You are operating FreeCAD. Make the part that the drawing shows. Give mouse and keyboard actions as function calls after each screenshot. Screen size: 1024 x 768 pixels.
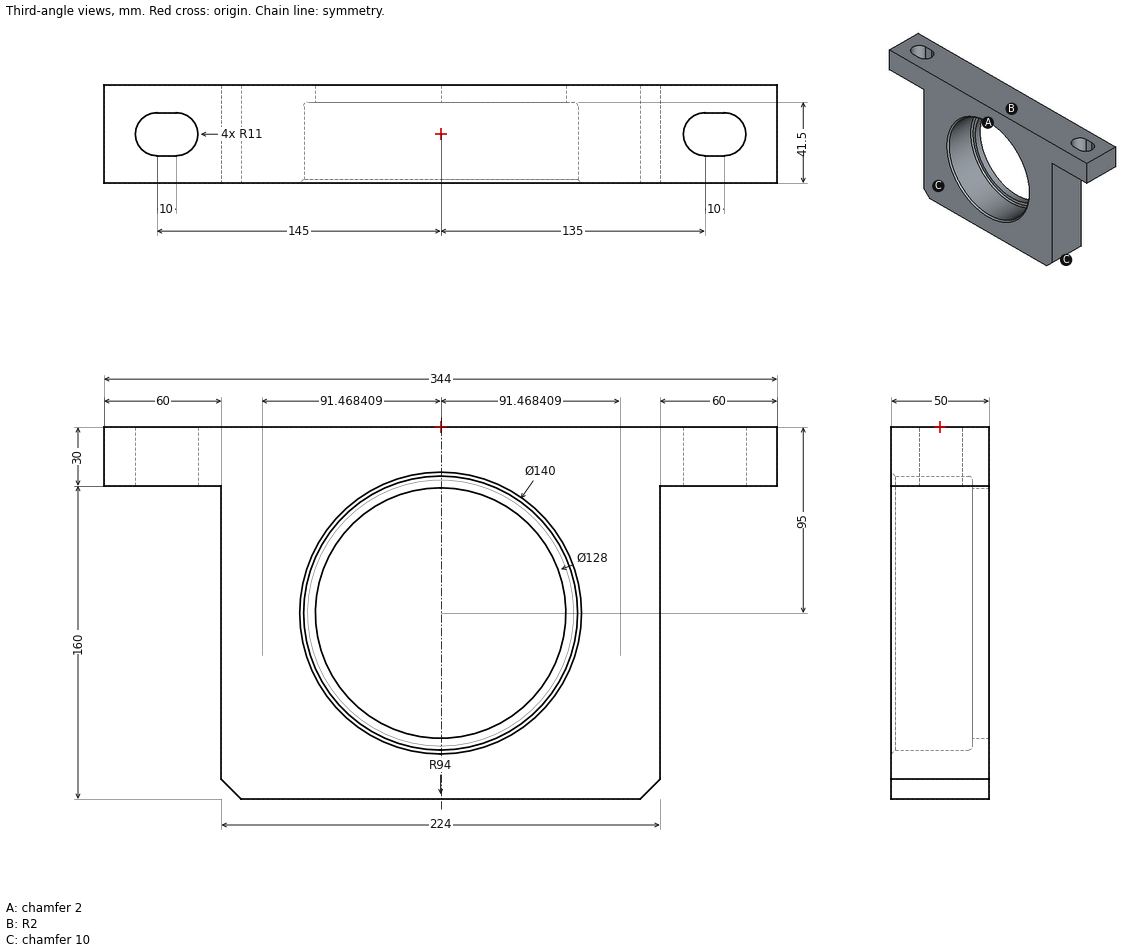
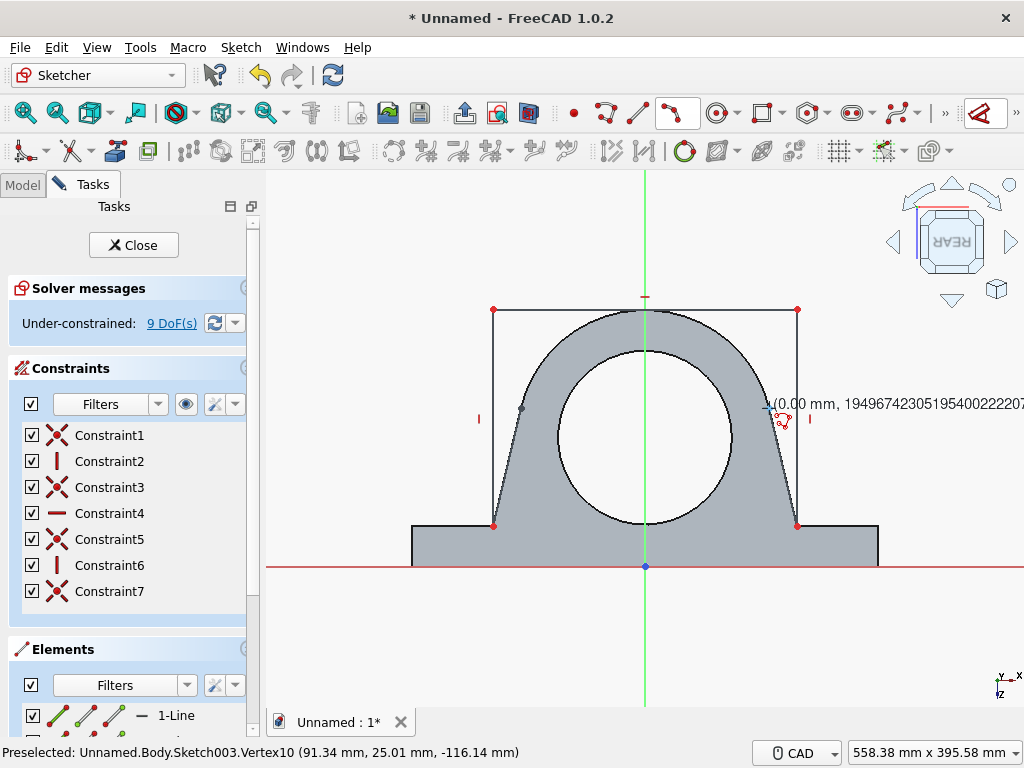
key(g)
key(3)
key(a)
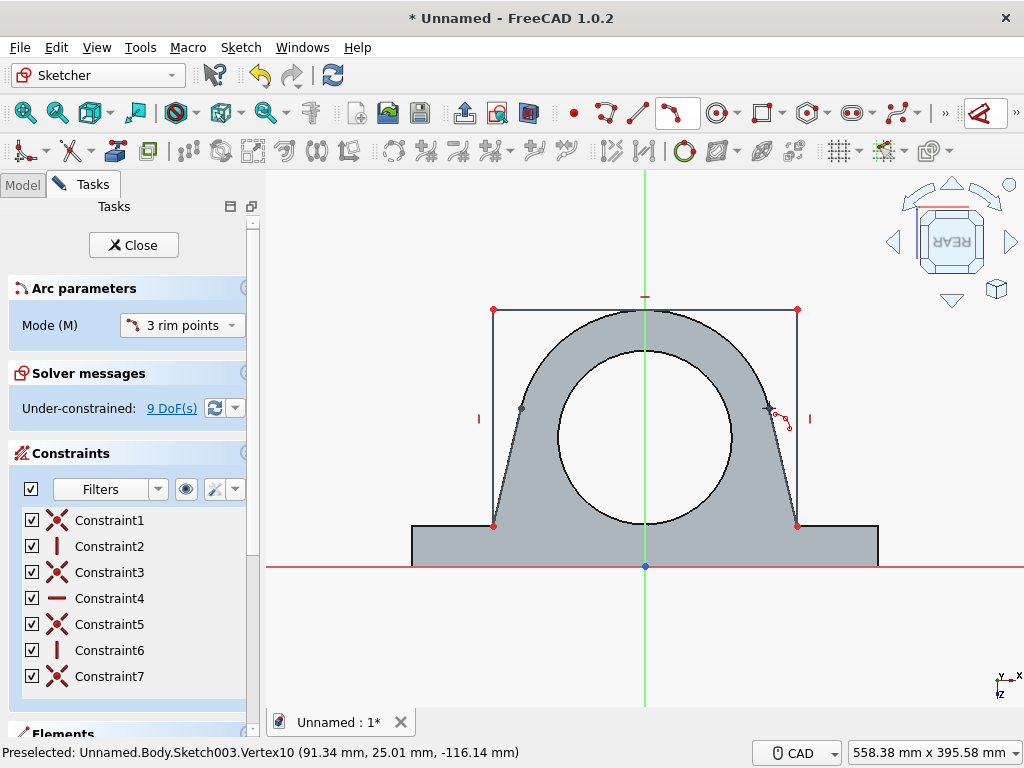
click(769, 409)
click(521, 409)
click(710, 328)
key(Escape)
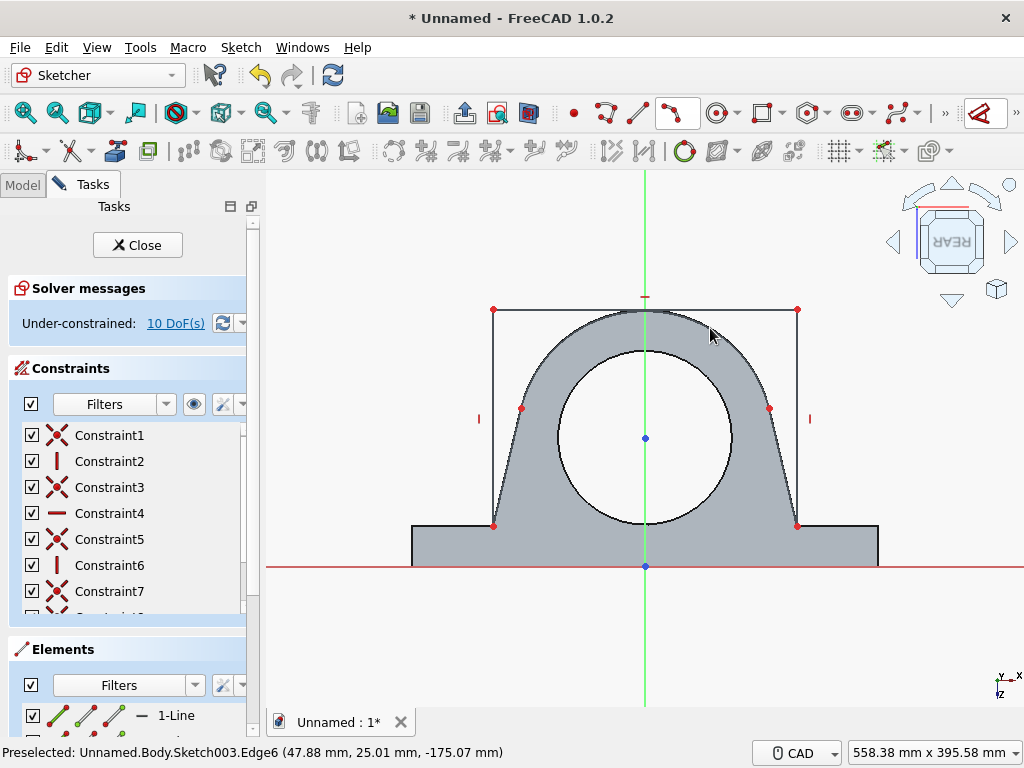
click(645, 439)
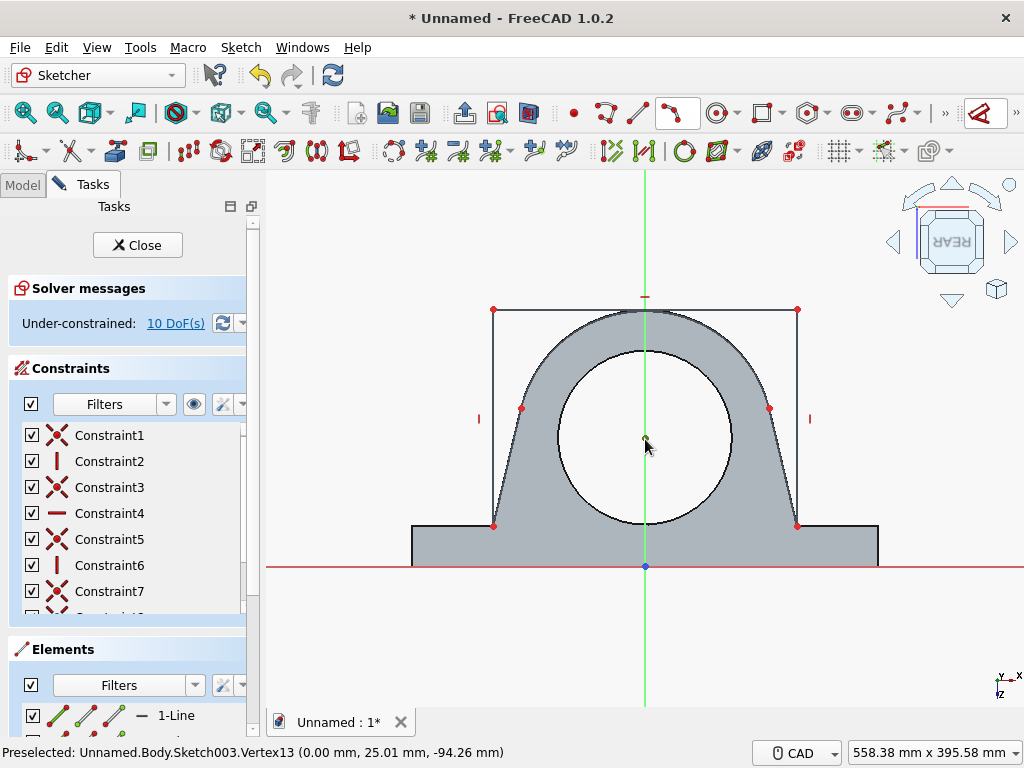
click(645, 645)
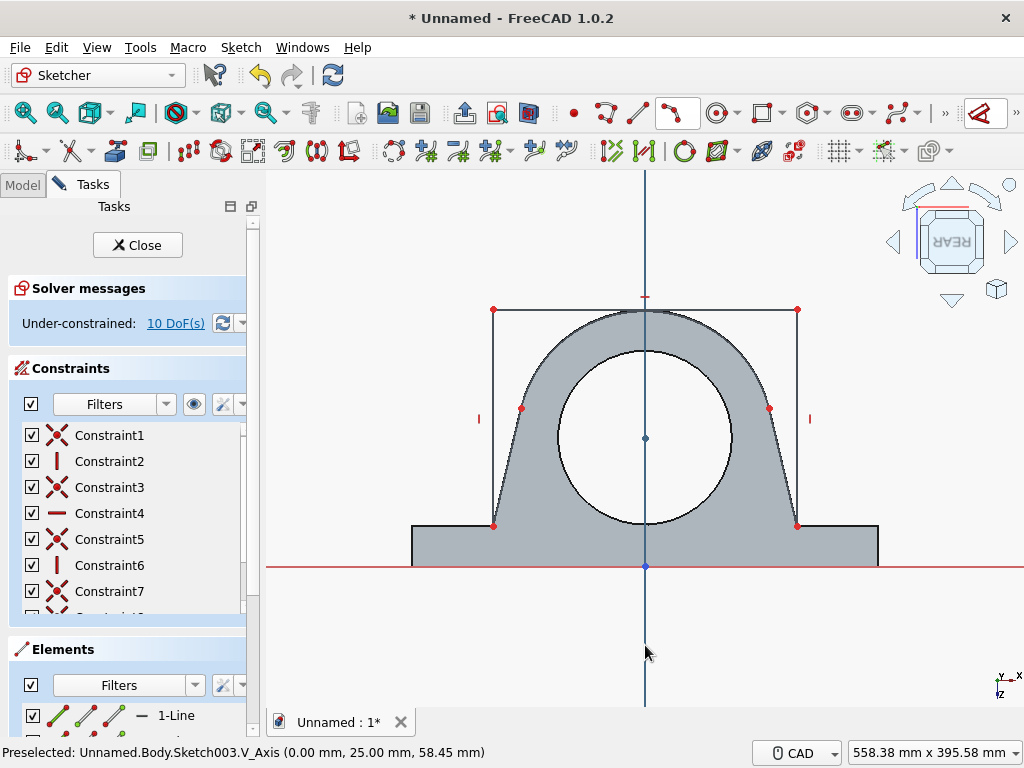
key(c)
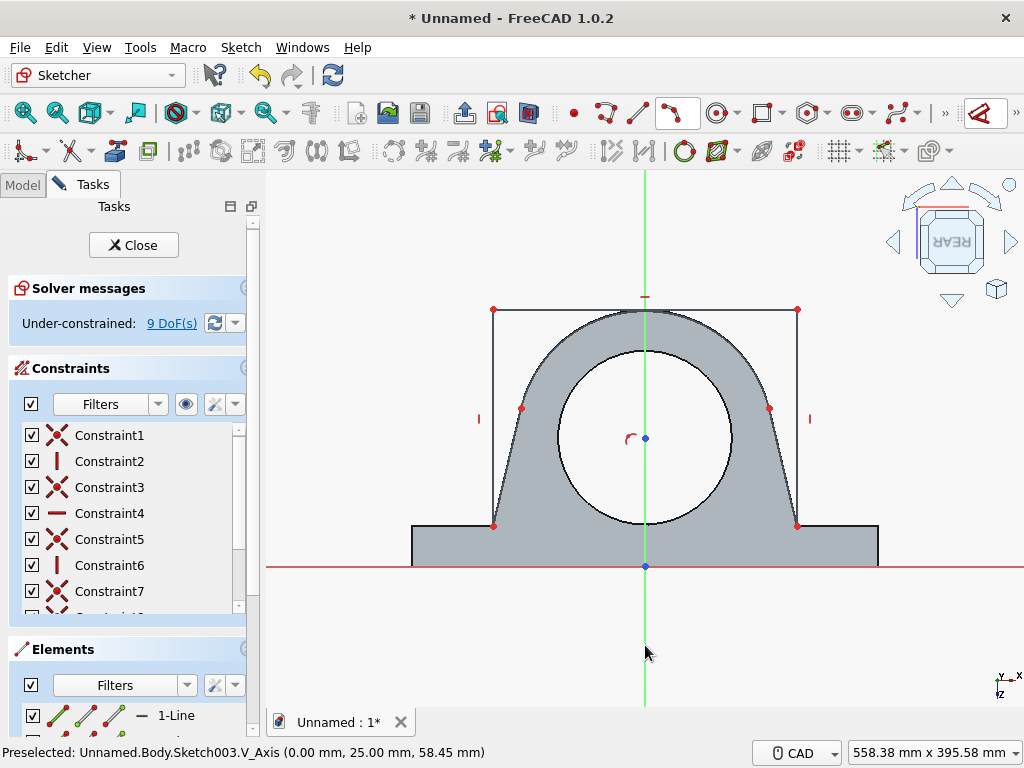
click(493, 527)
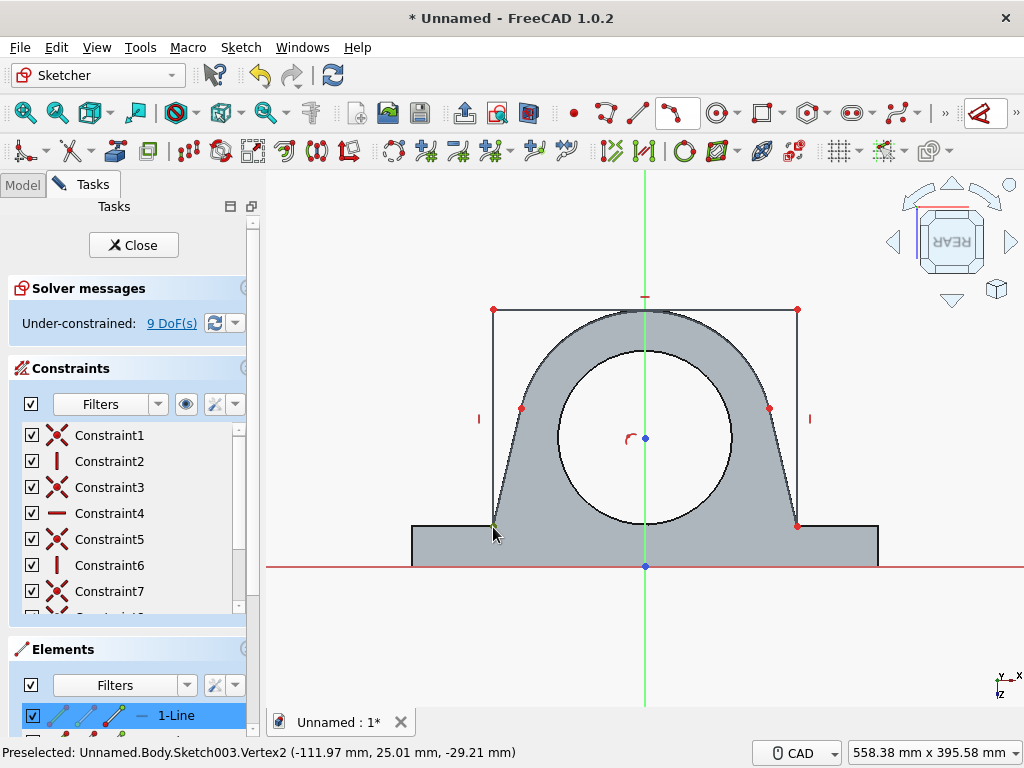
click(797, 527)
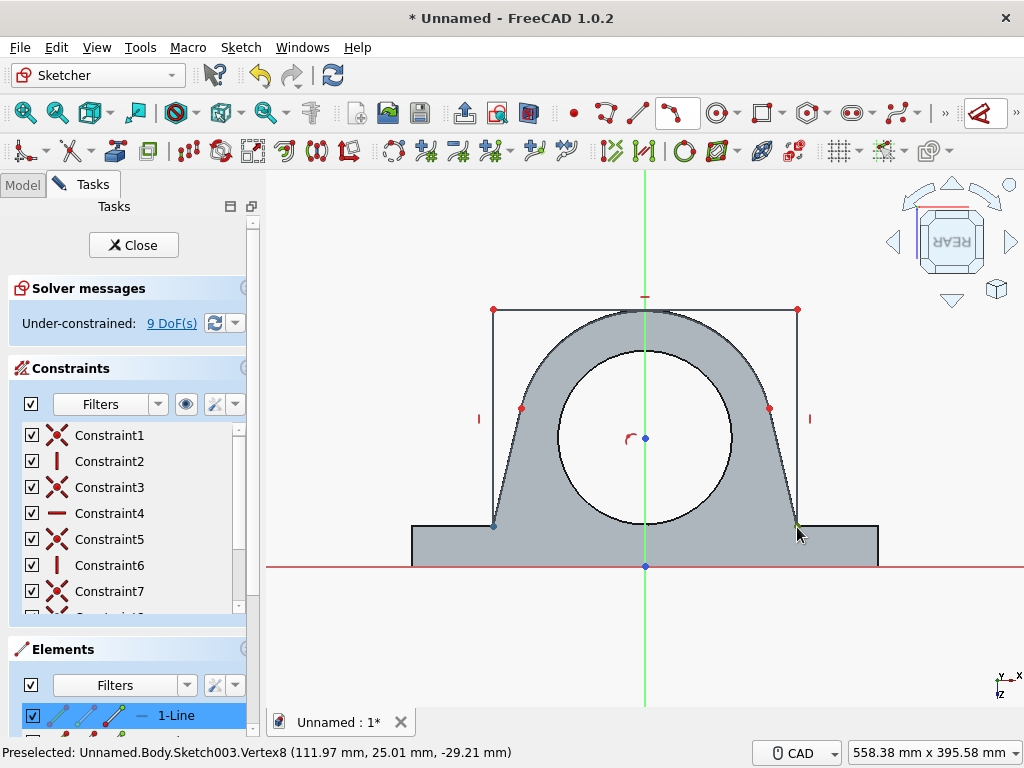
click(645, 645)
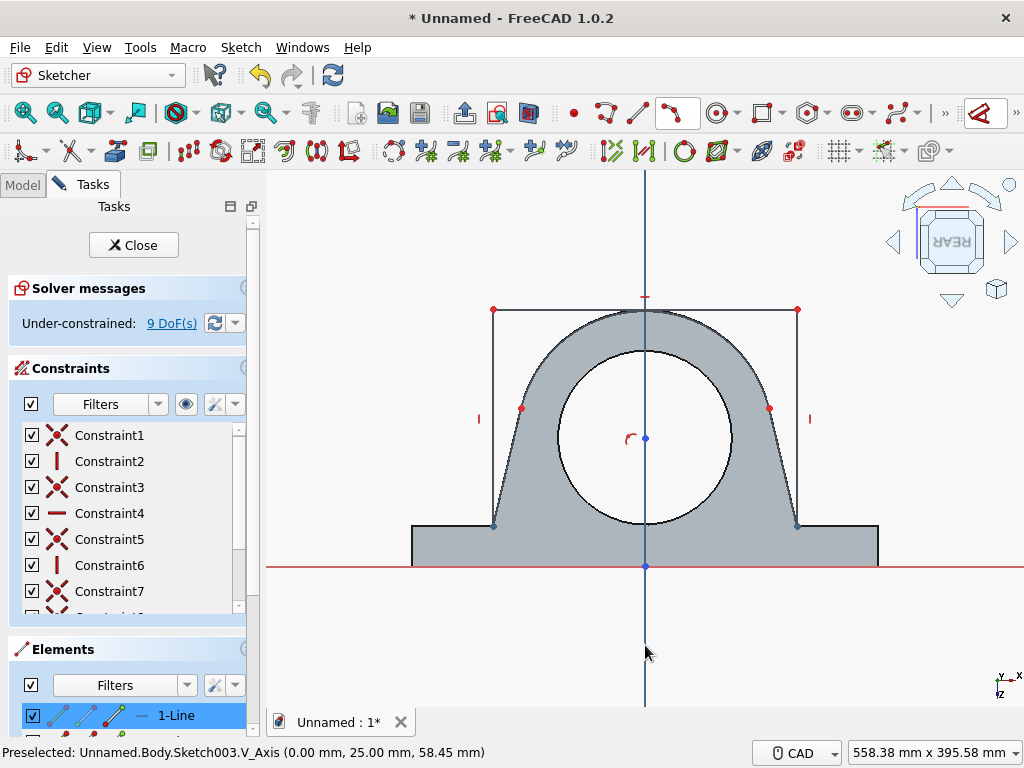
key(s)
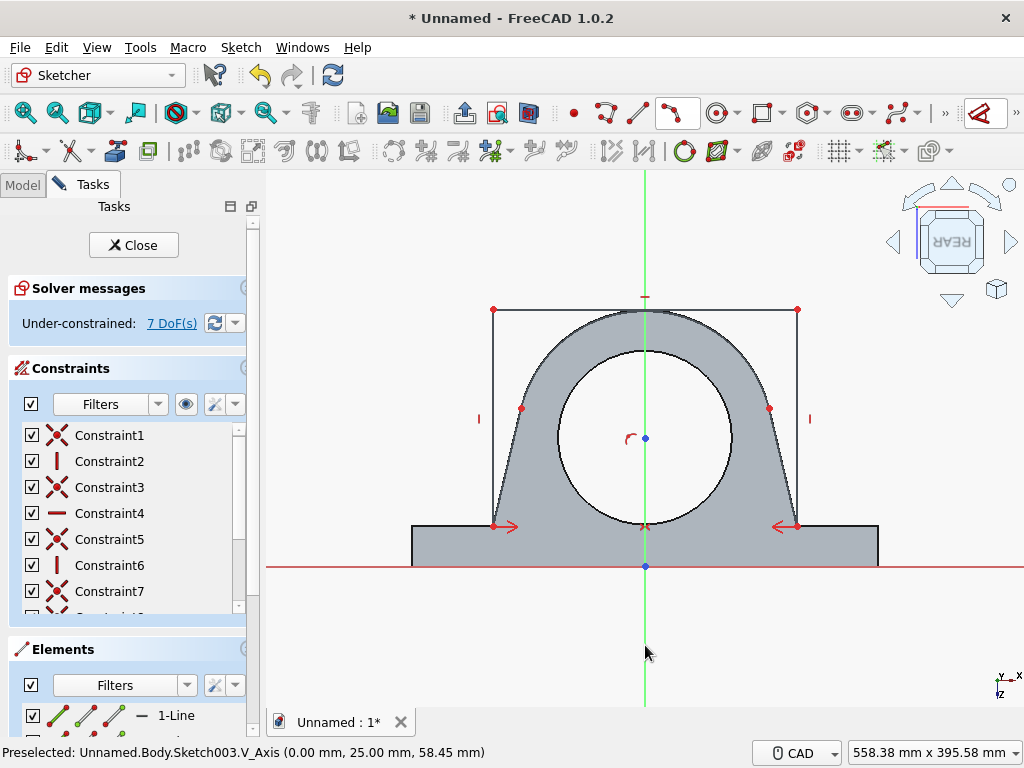
key(d)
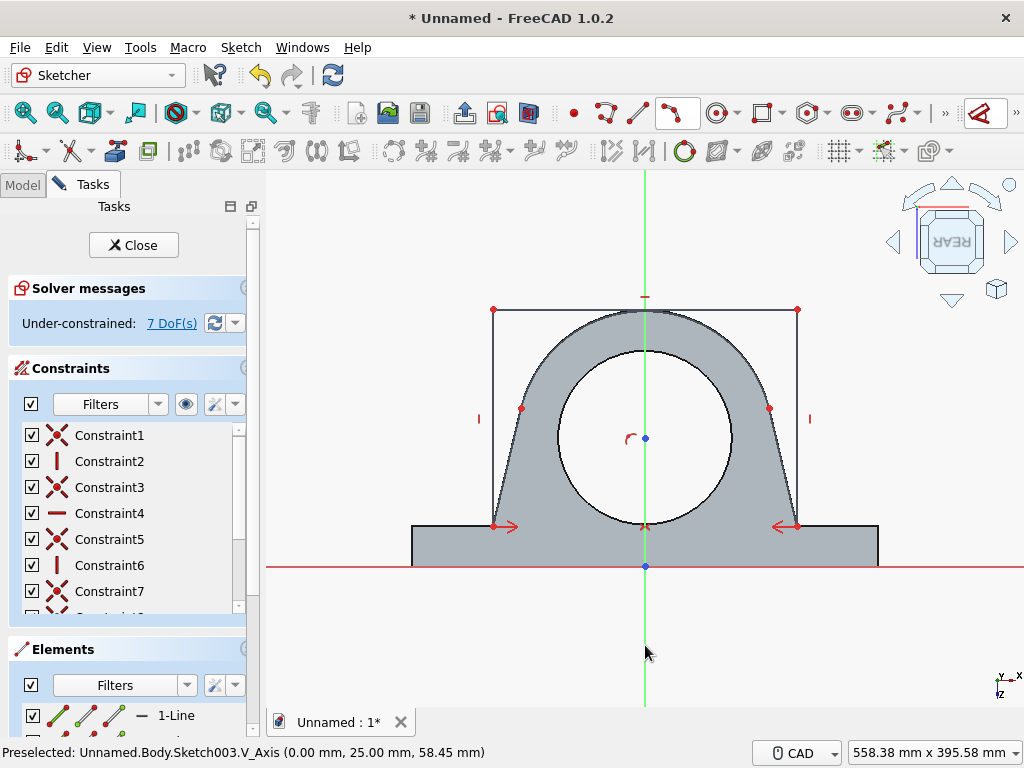
click(710, 329)
click(782, 357)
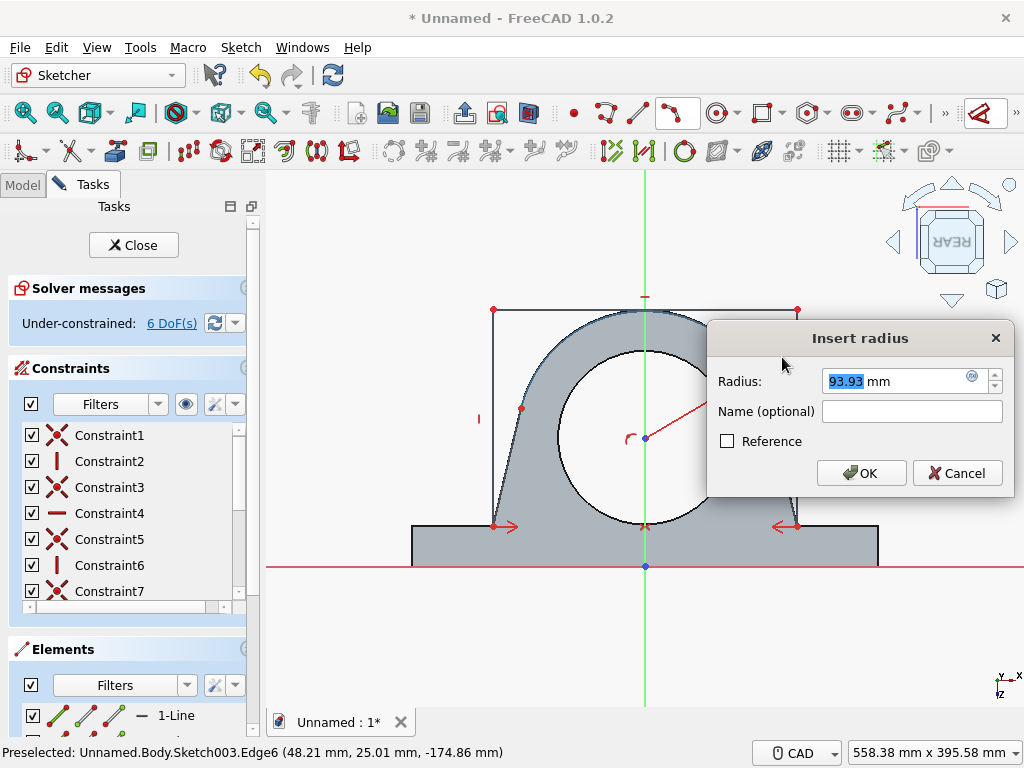
text(94)
key(Return)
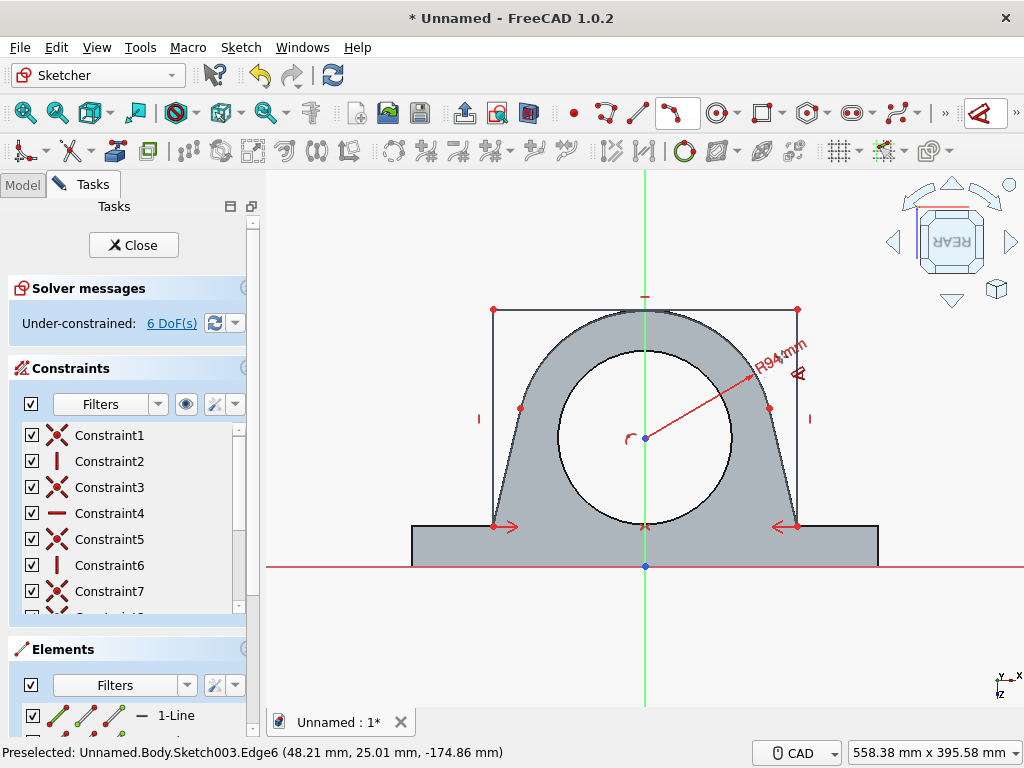
click(493, 462)
click(459, 418)